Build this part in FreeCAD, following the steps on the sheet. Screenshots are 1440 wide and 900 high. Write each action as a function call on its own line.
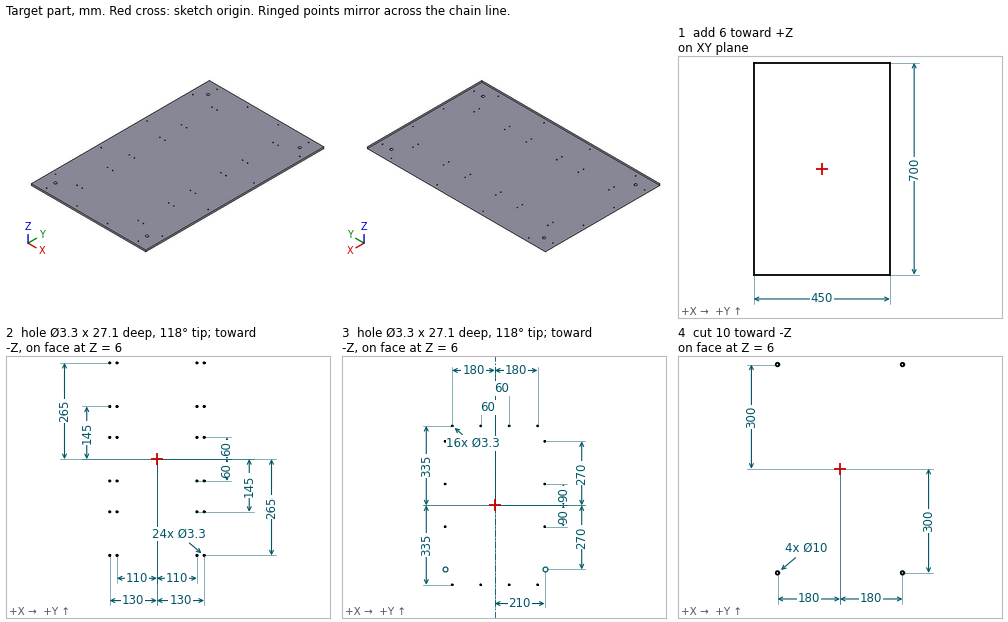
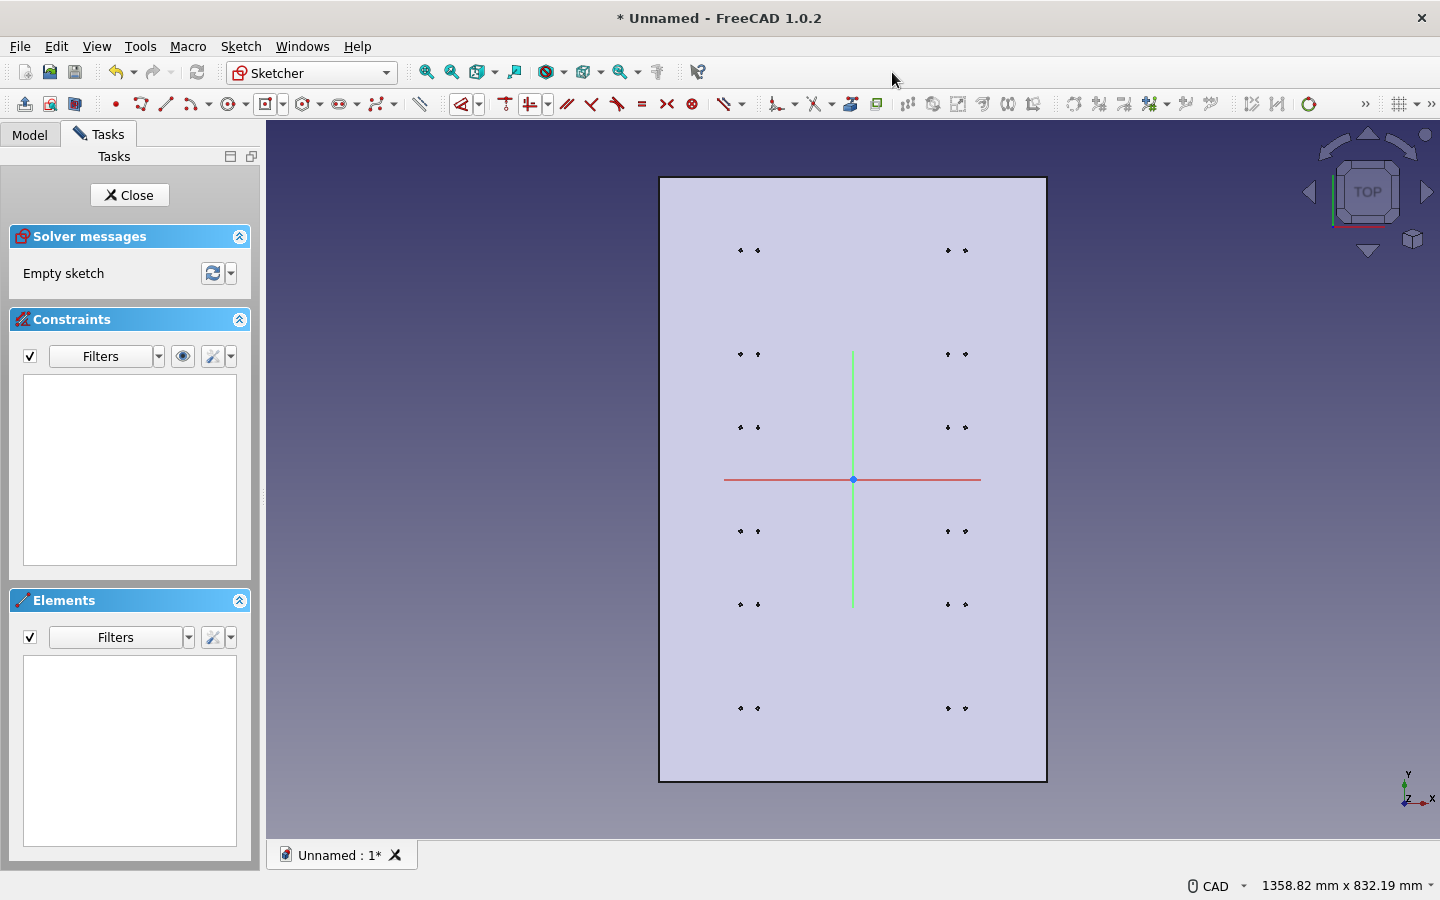
click(228, 104)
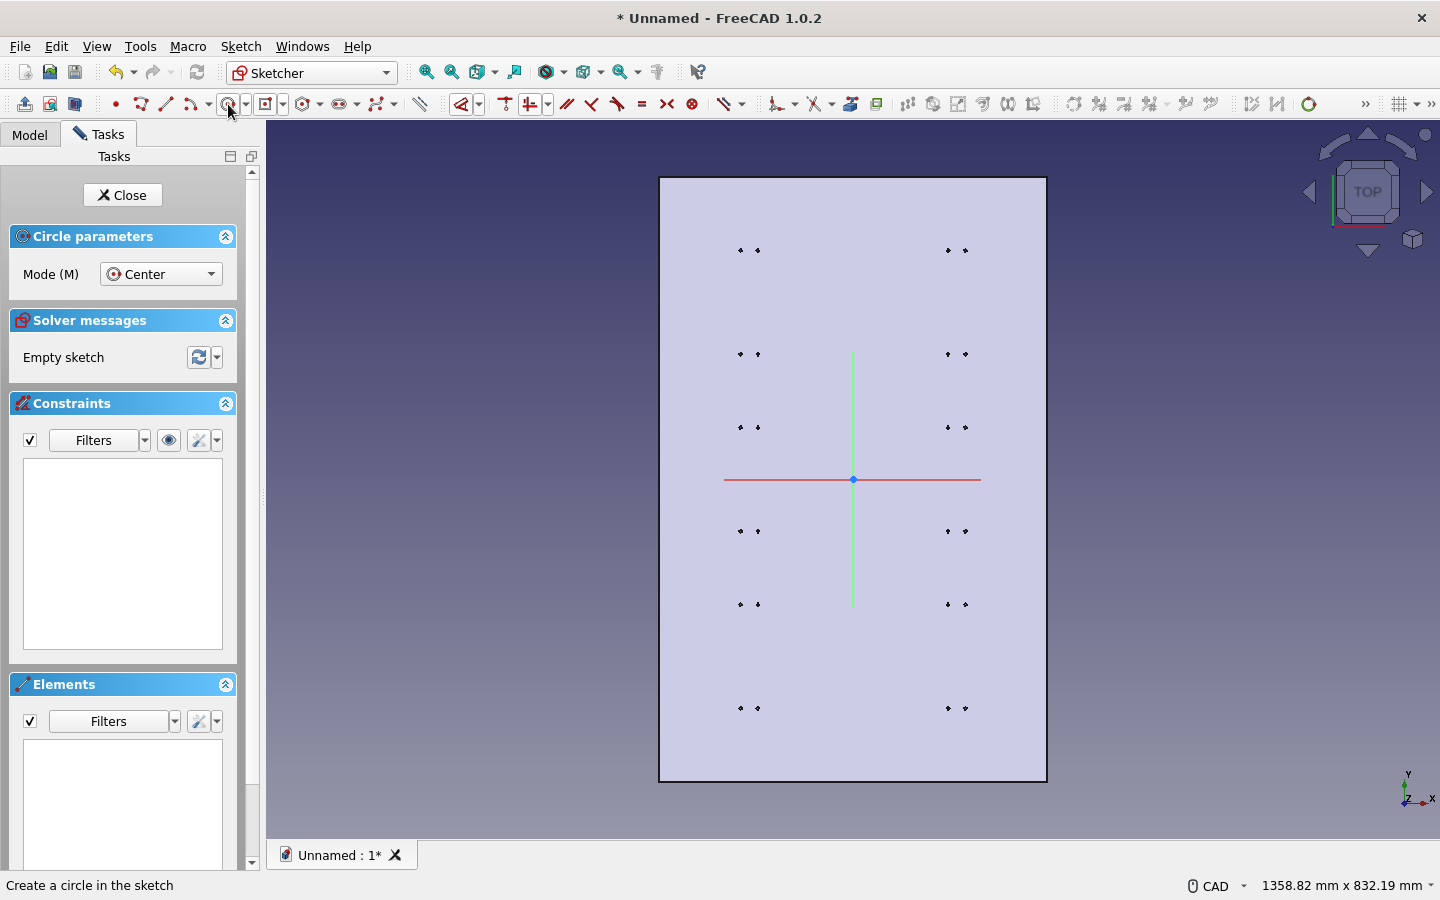
scroll(697, 190, up, 14)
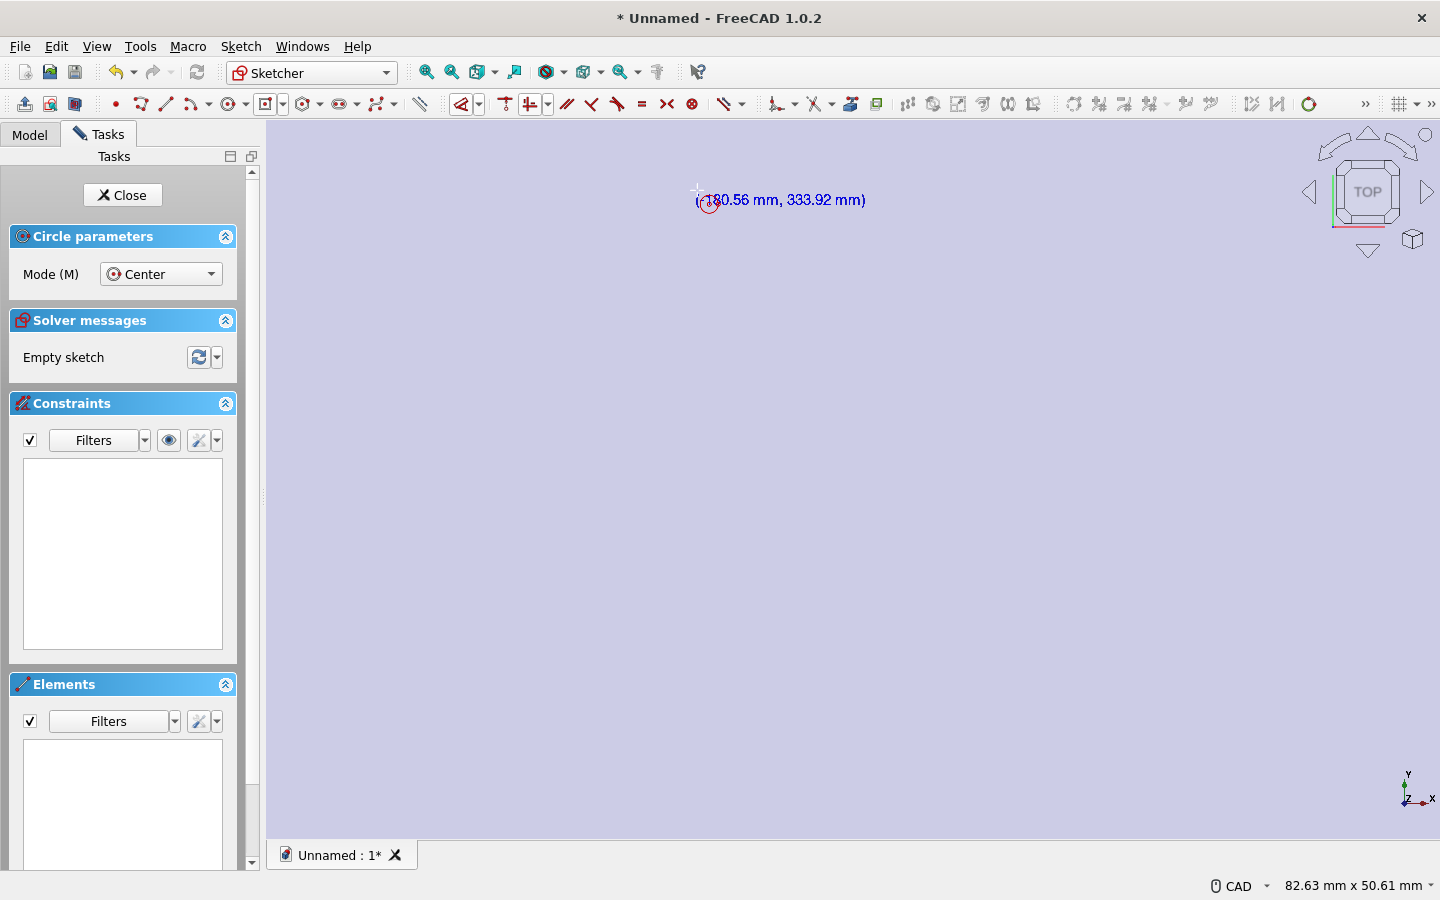
scroll(655, 245, down, 15)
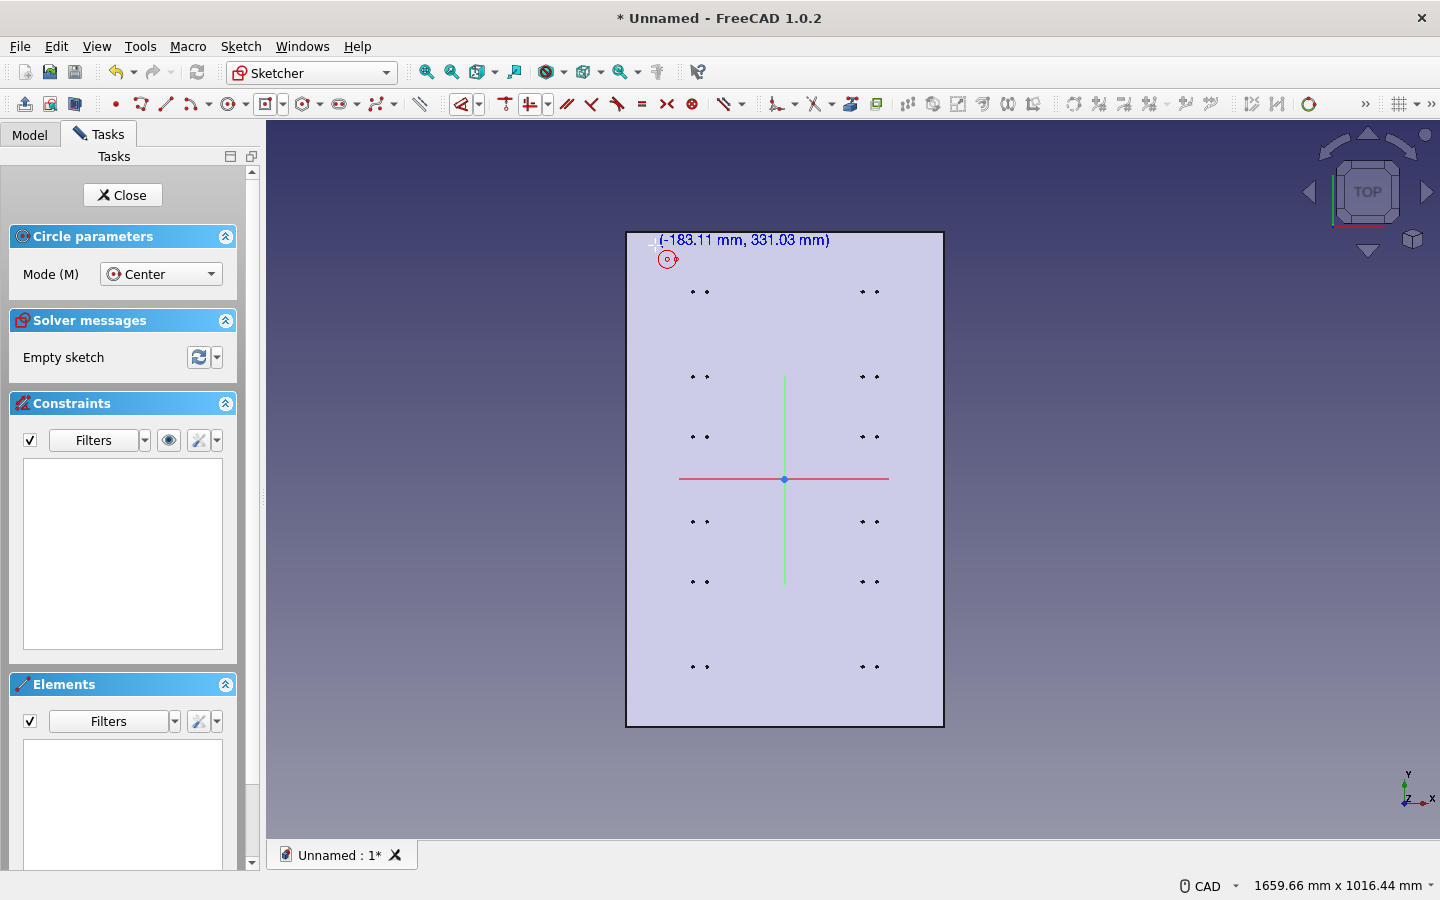
click(658, 242)
move(658, 242)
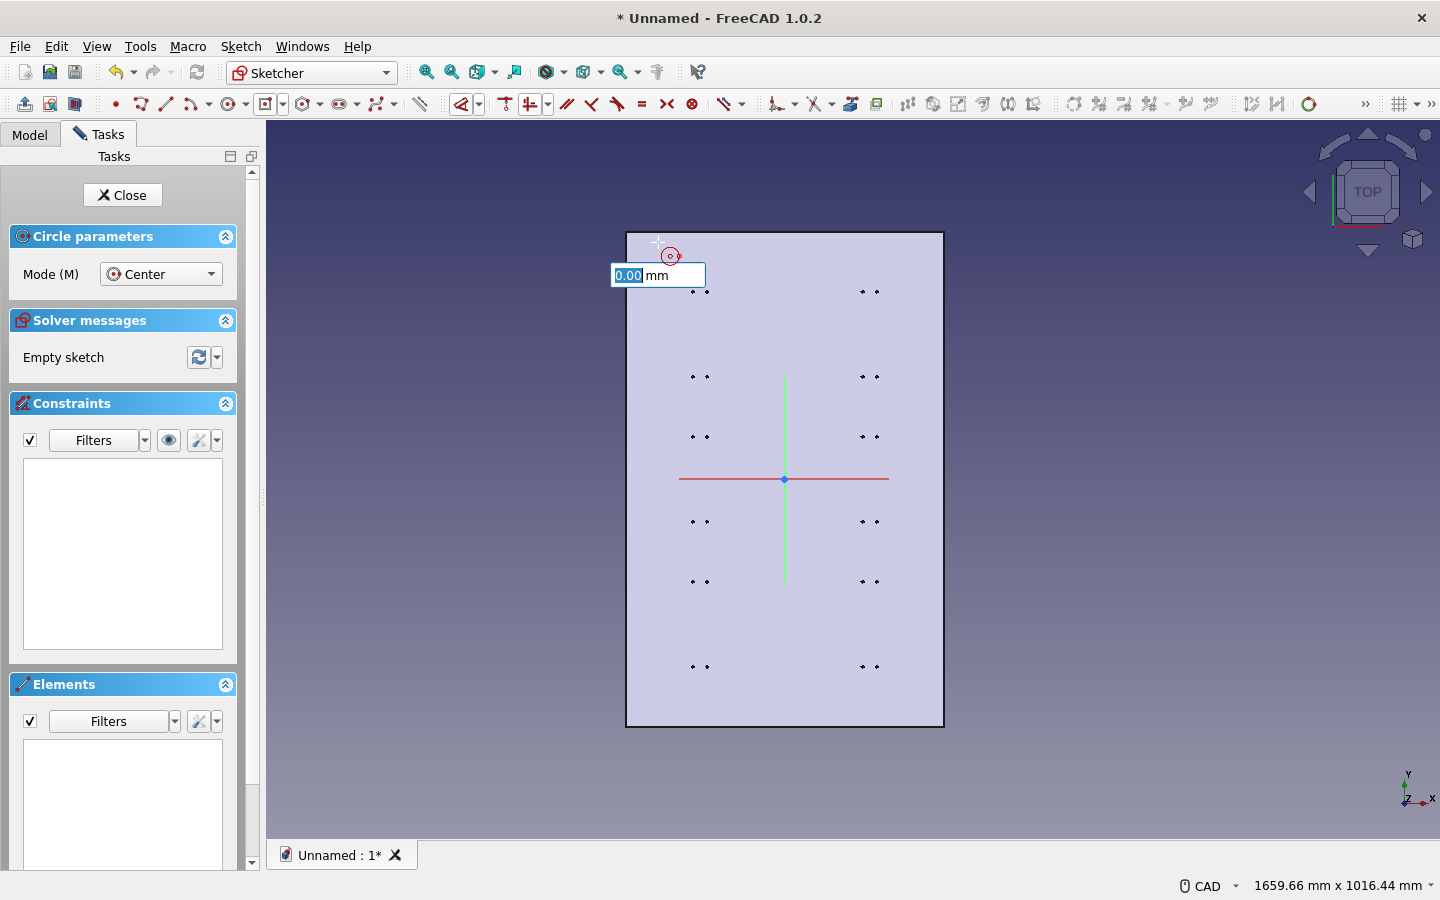
text(3.3)
key(Return)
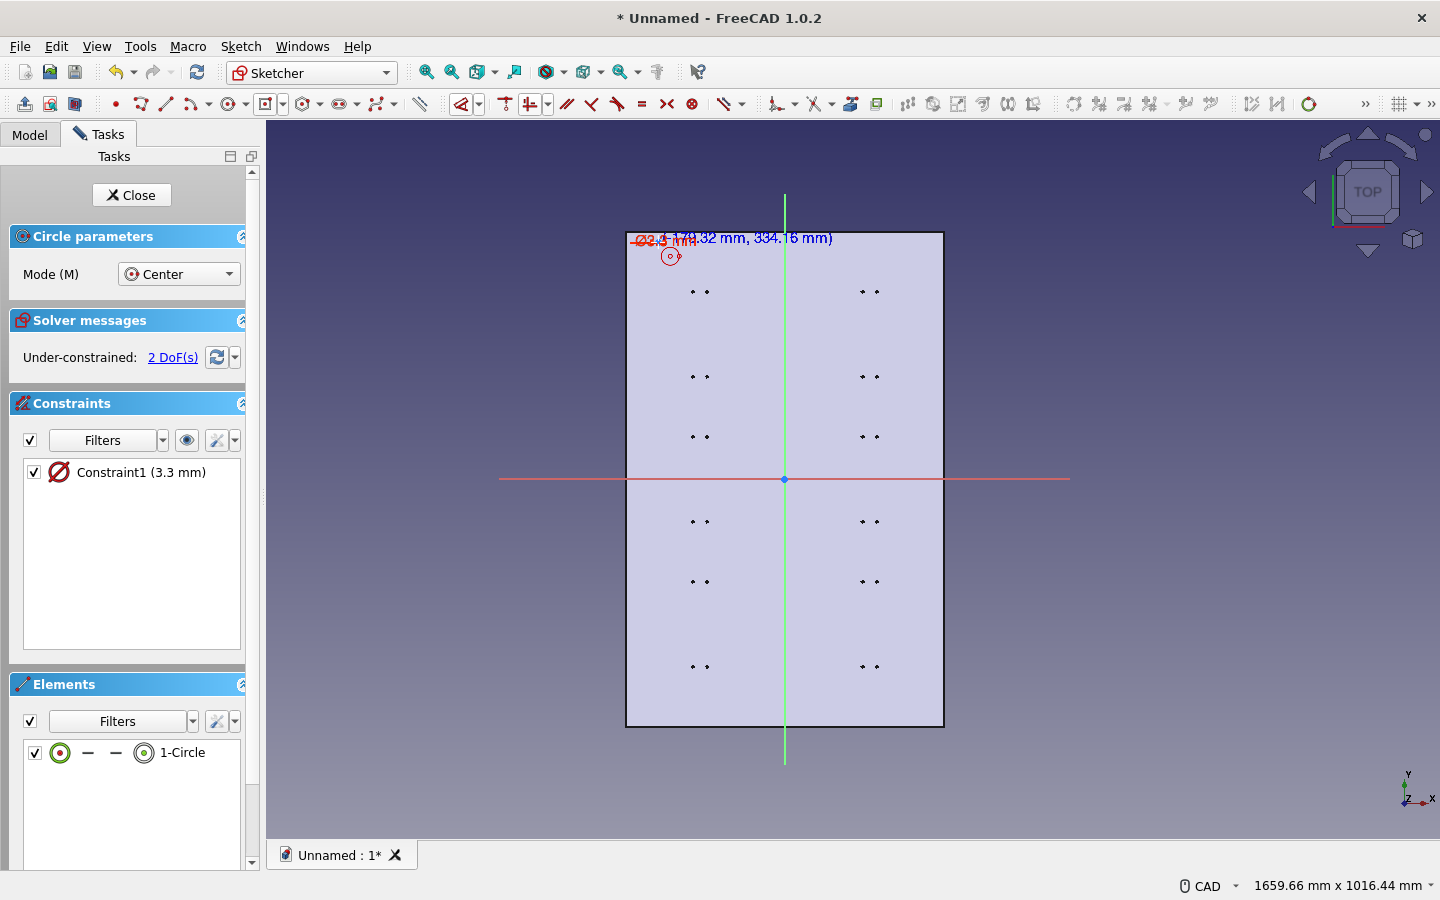
scroll(742, 242, up, 15)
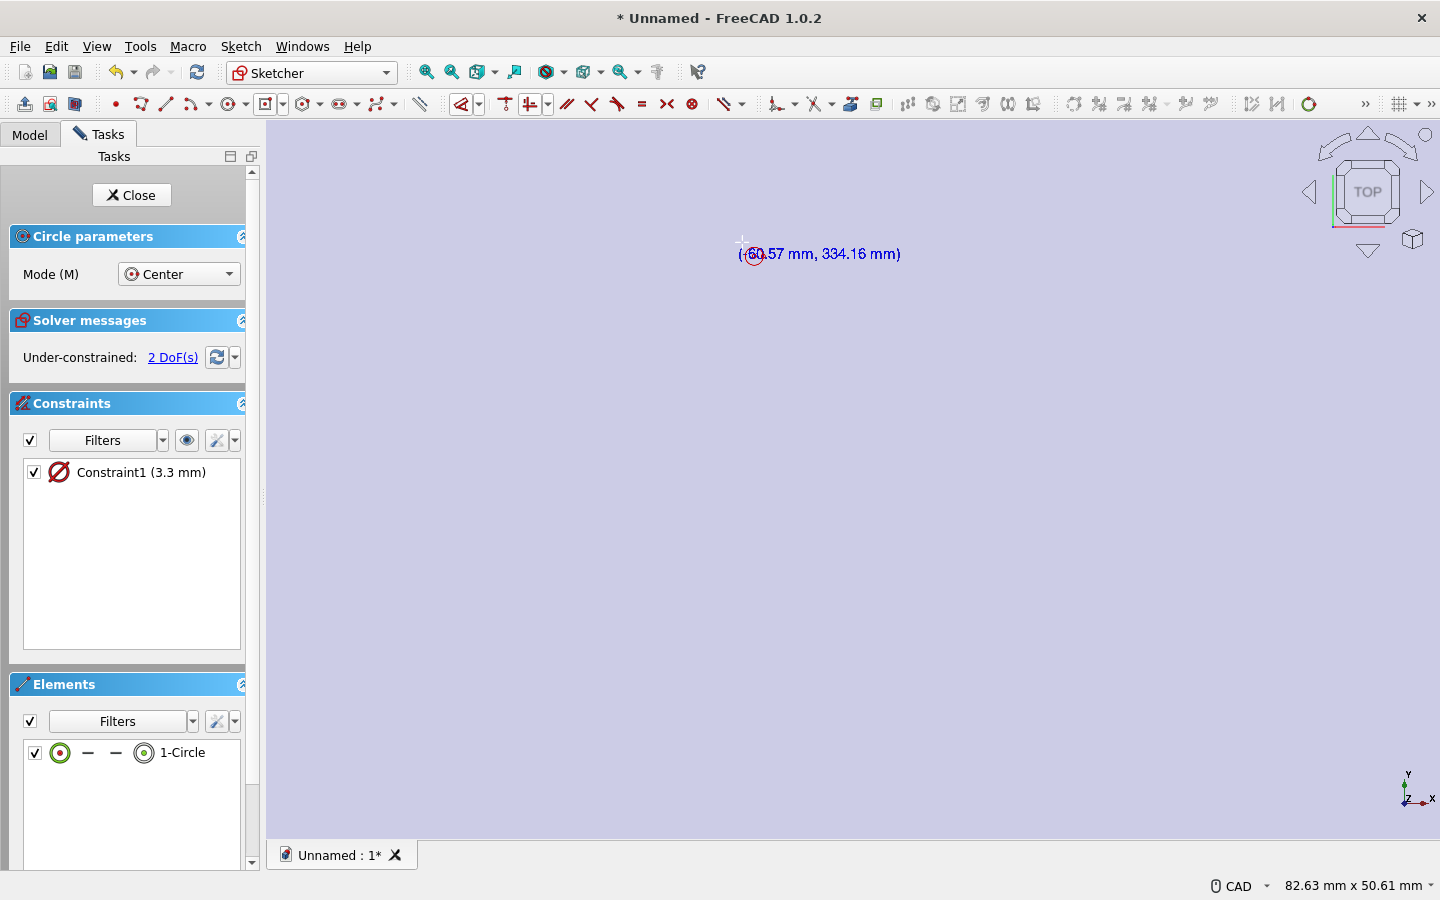
scroll(742, 242, down, 15)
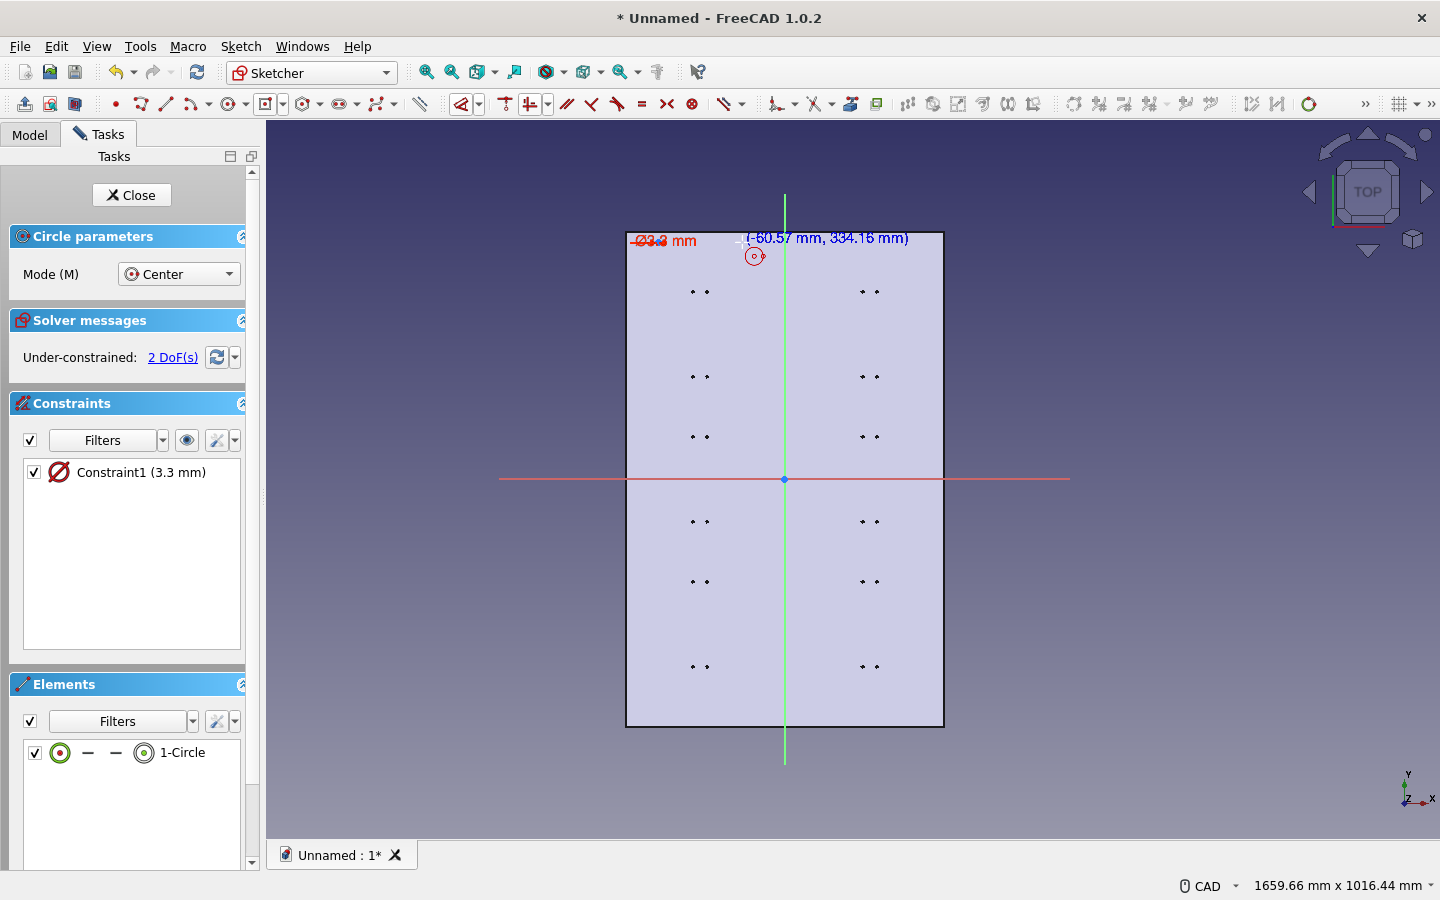
click(742, 242)
move(743, 242)